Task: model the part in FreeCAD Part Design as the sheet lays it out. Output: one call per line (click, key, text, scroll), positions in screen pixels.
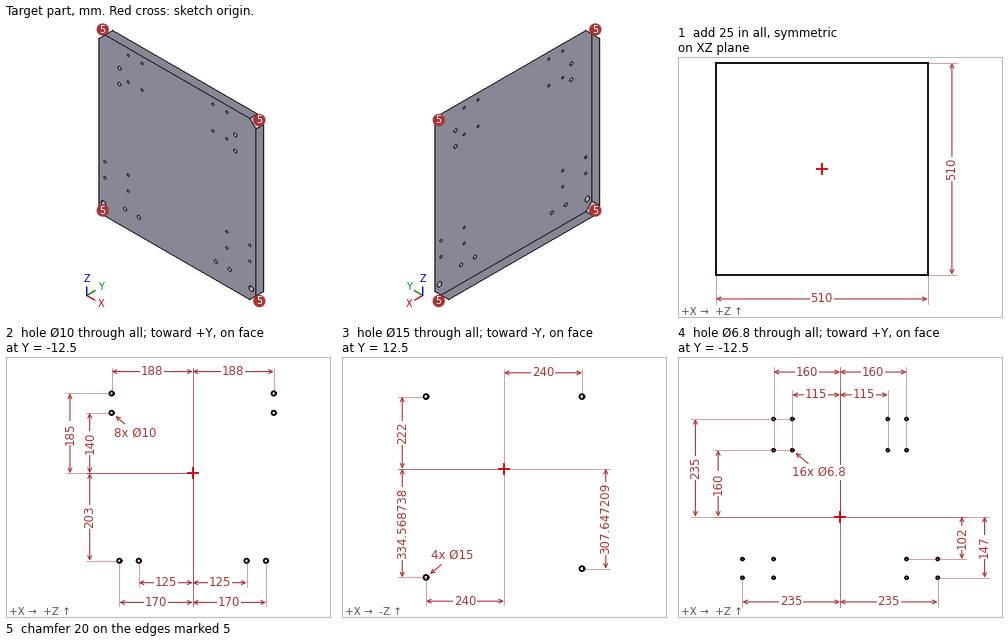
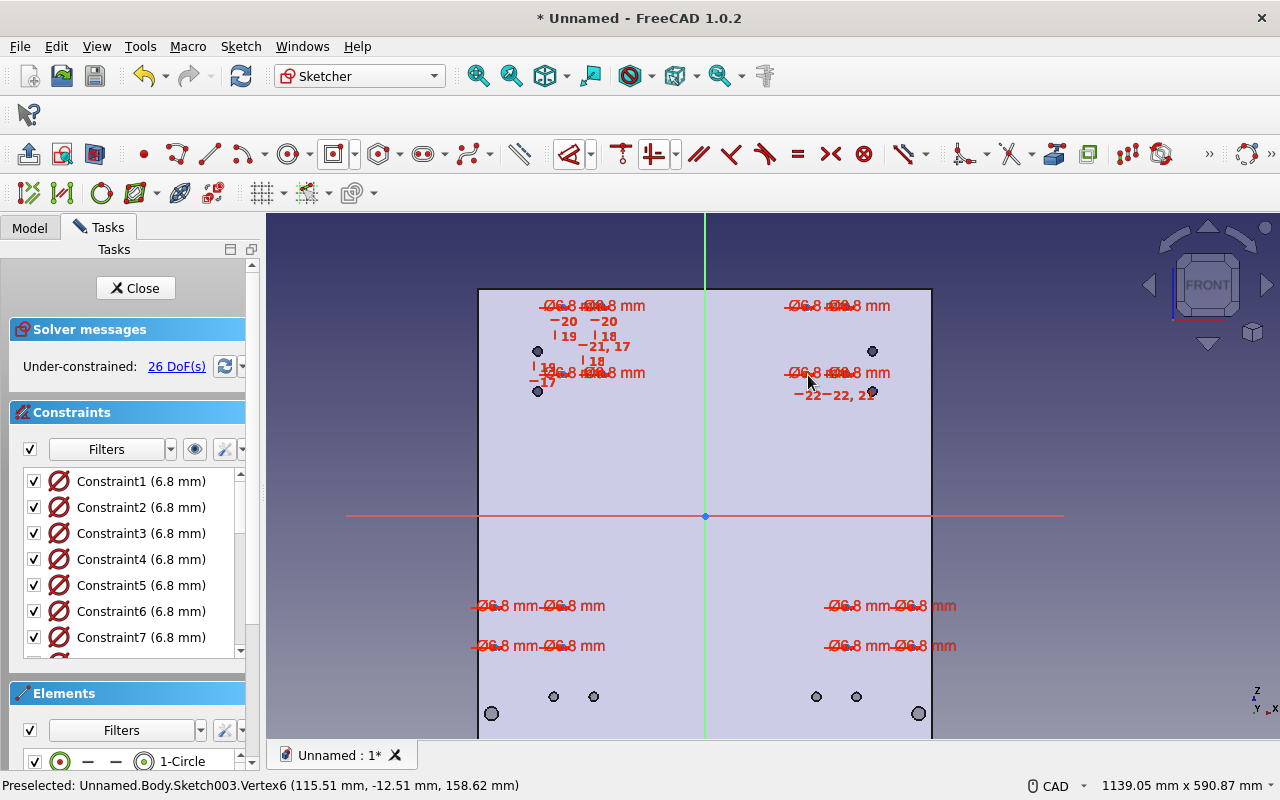
click(808, 308)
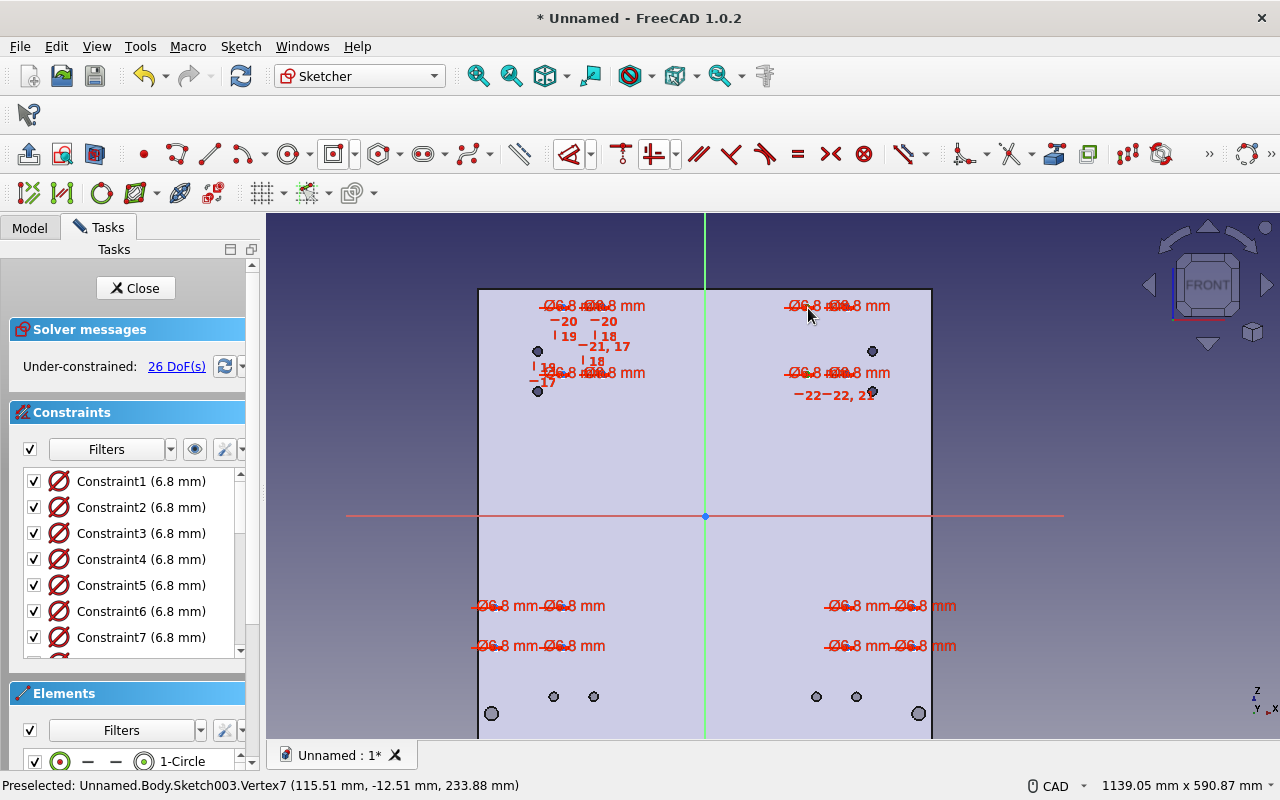
key(v)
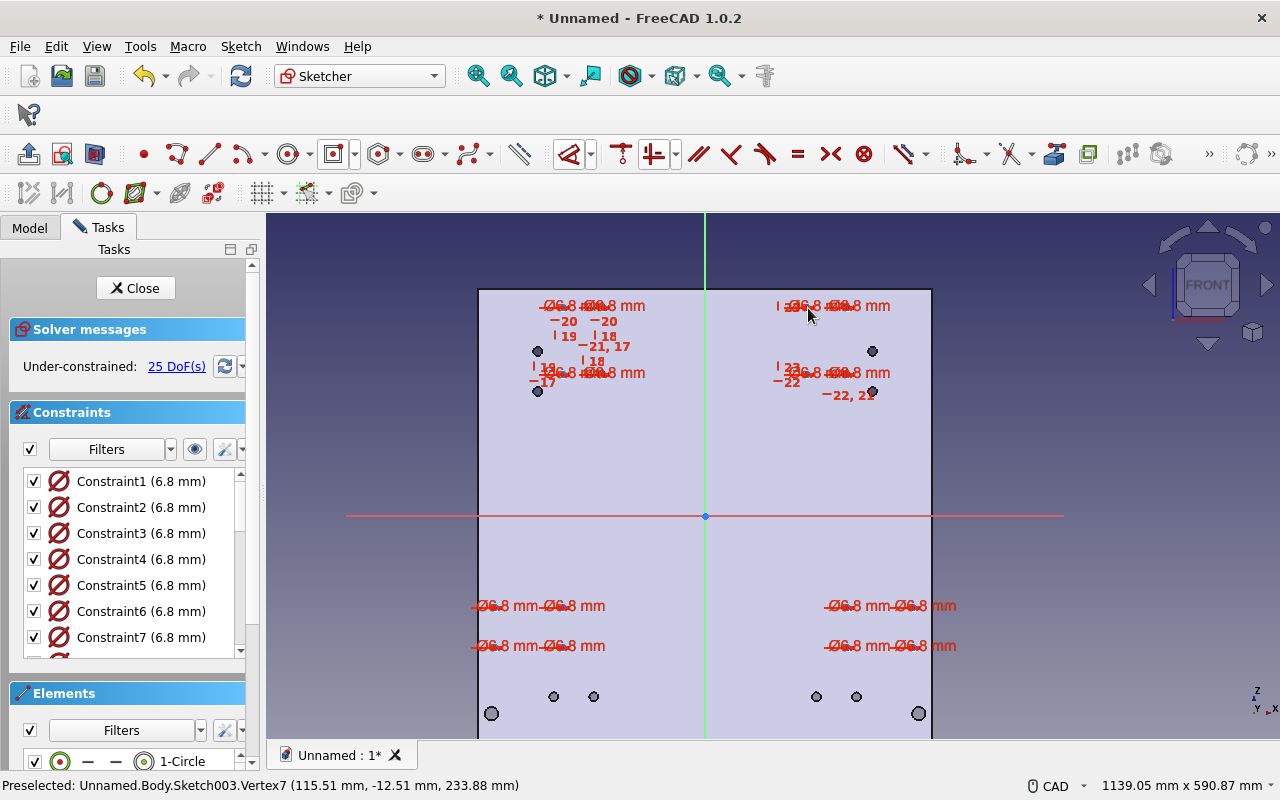
click(603, 308)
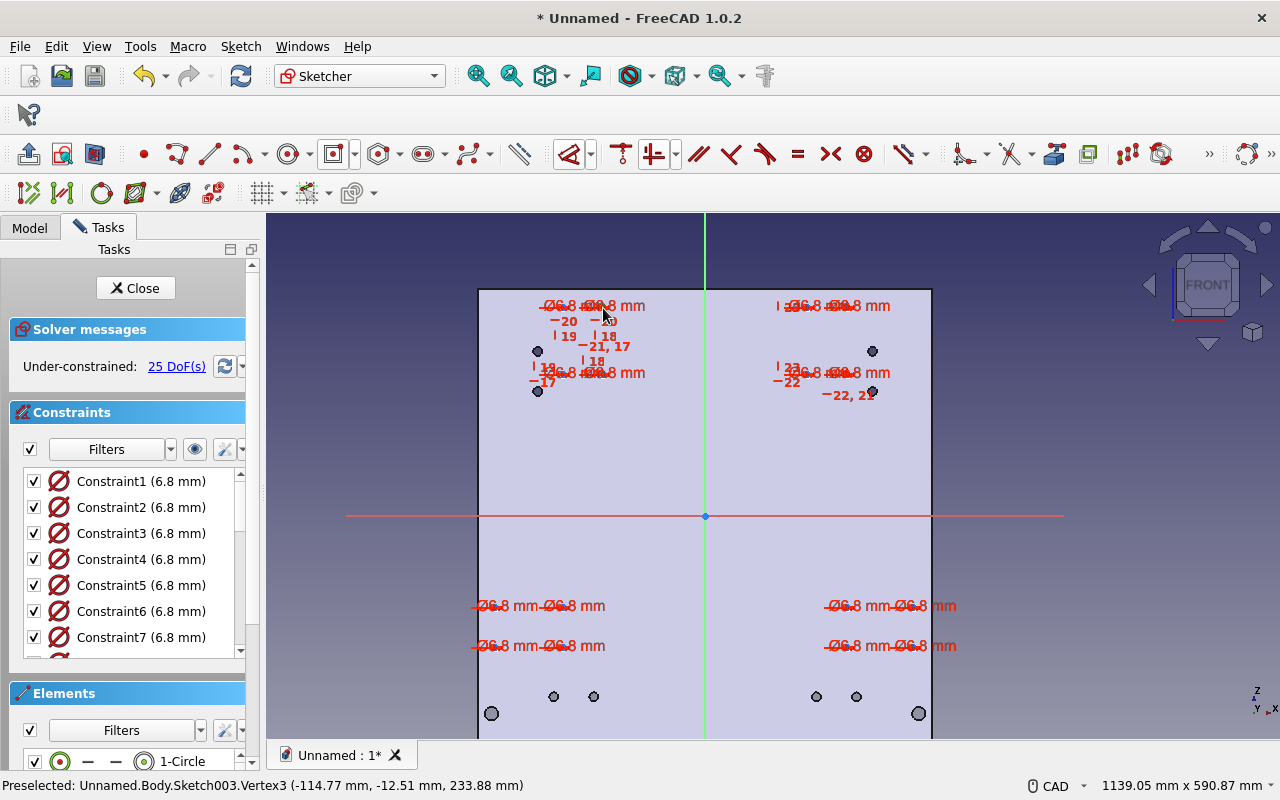
click(808, 308)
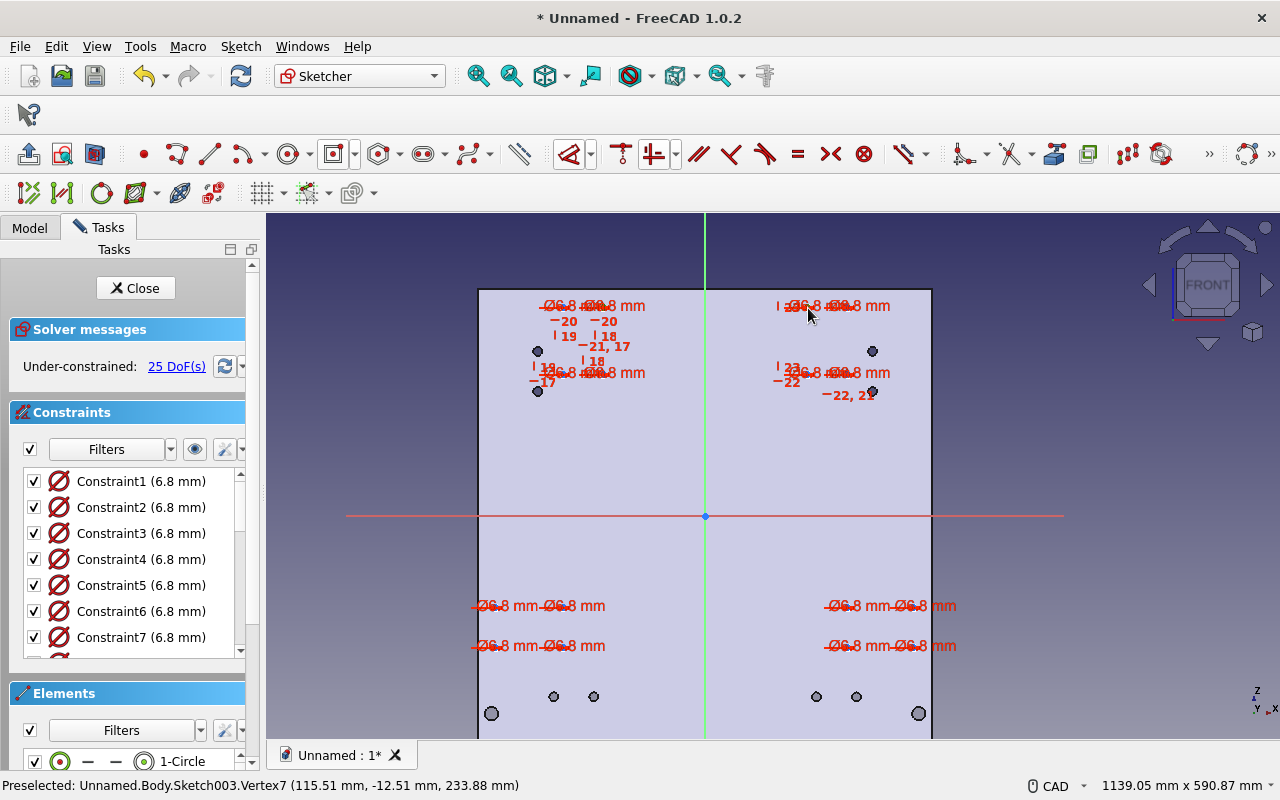
key(h)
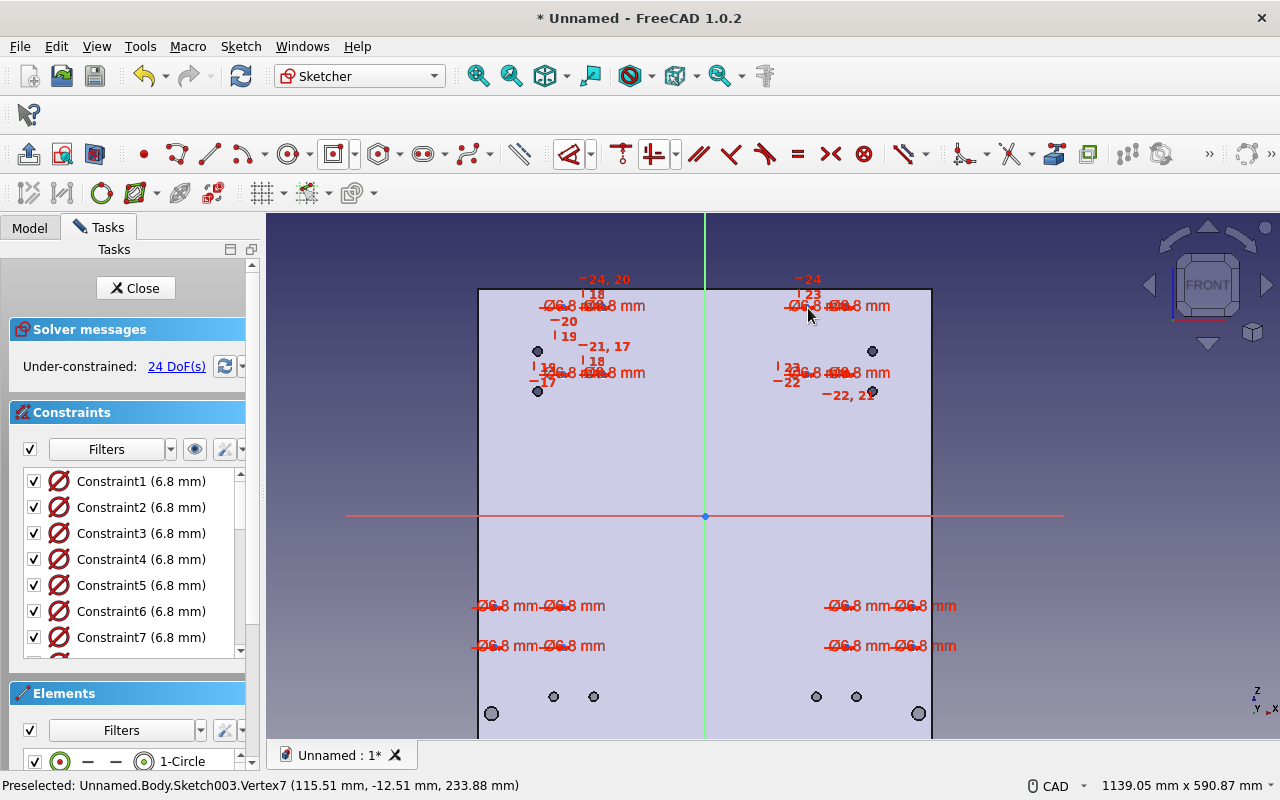
click(848, 375)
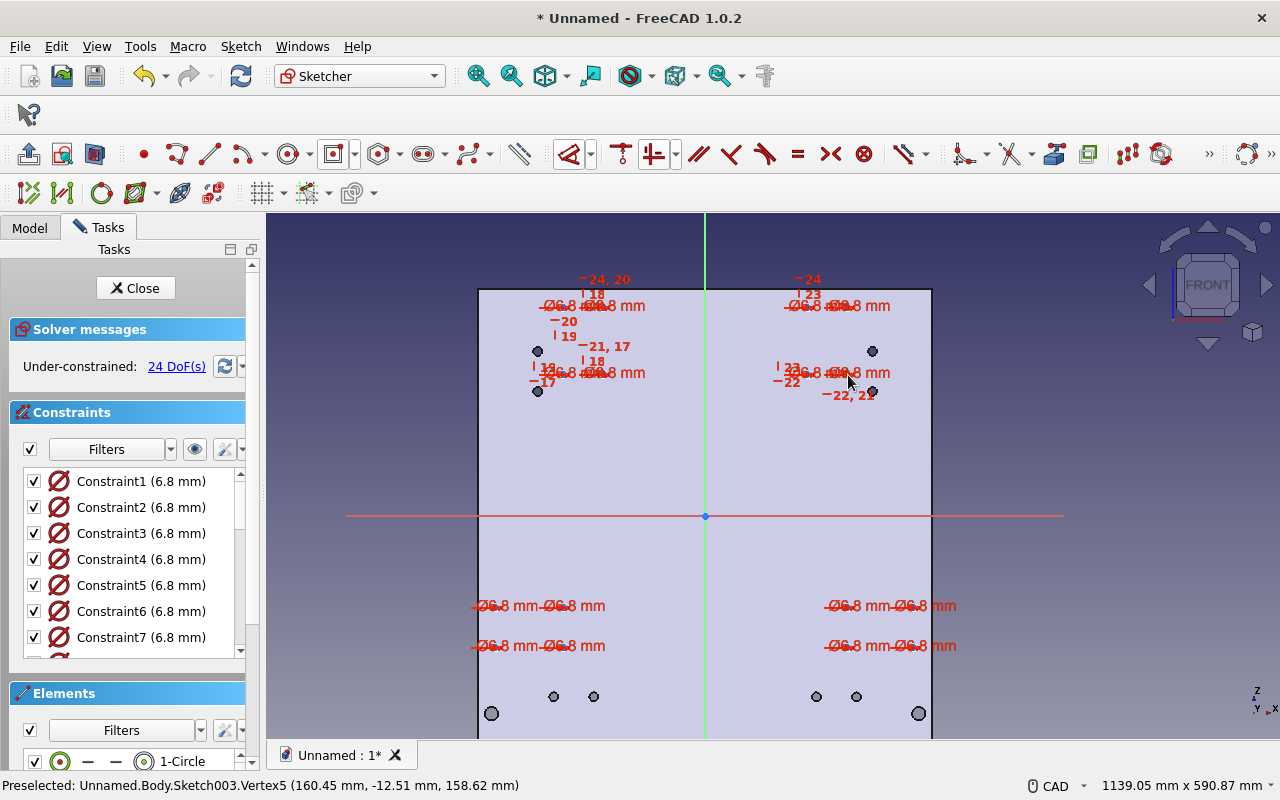
click(848, 308)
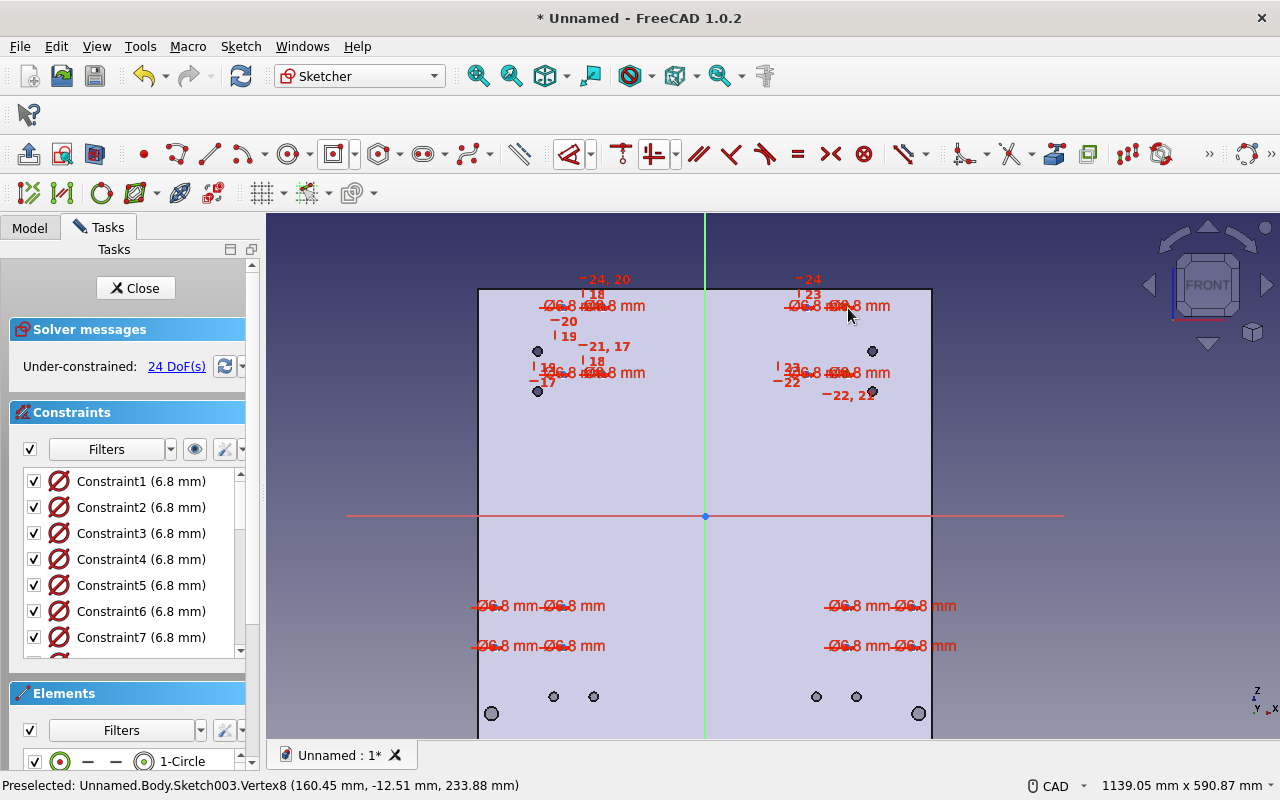
click(676, 154)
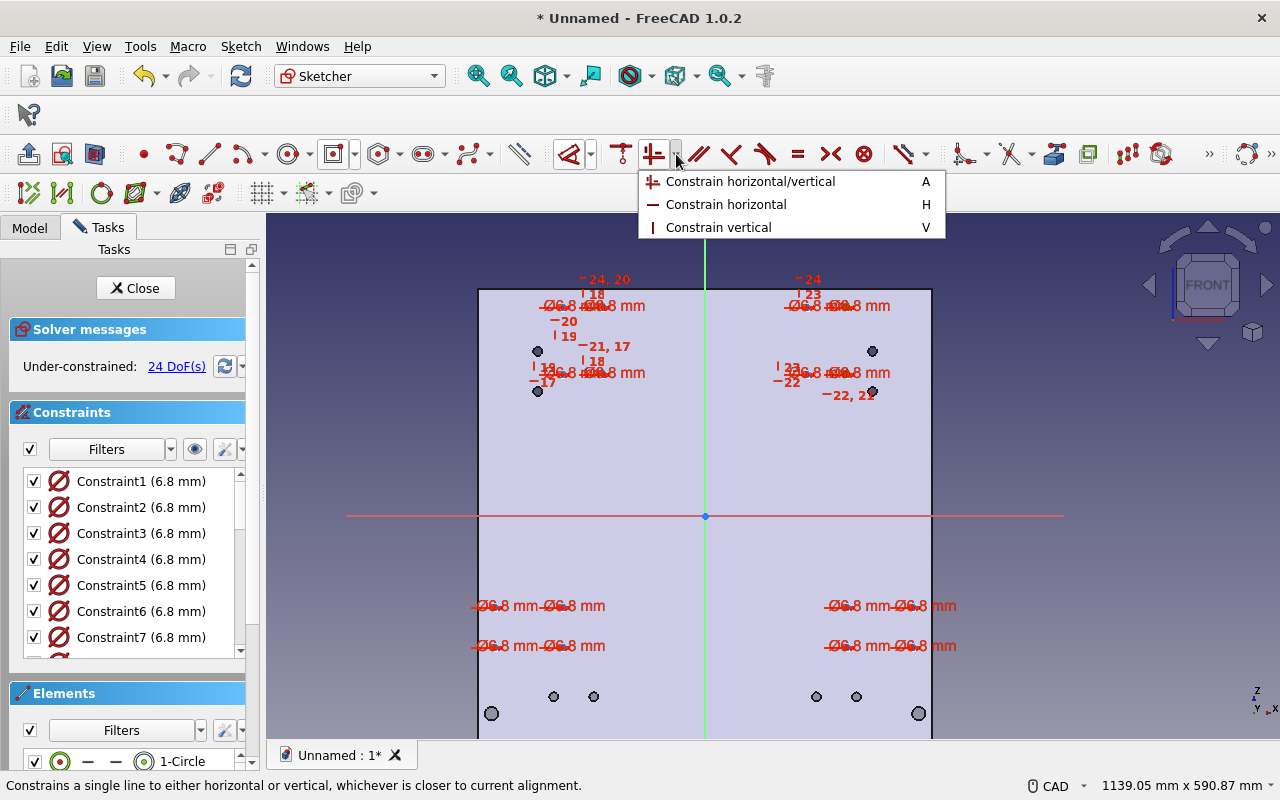
click(792, 228)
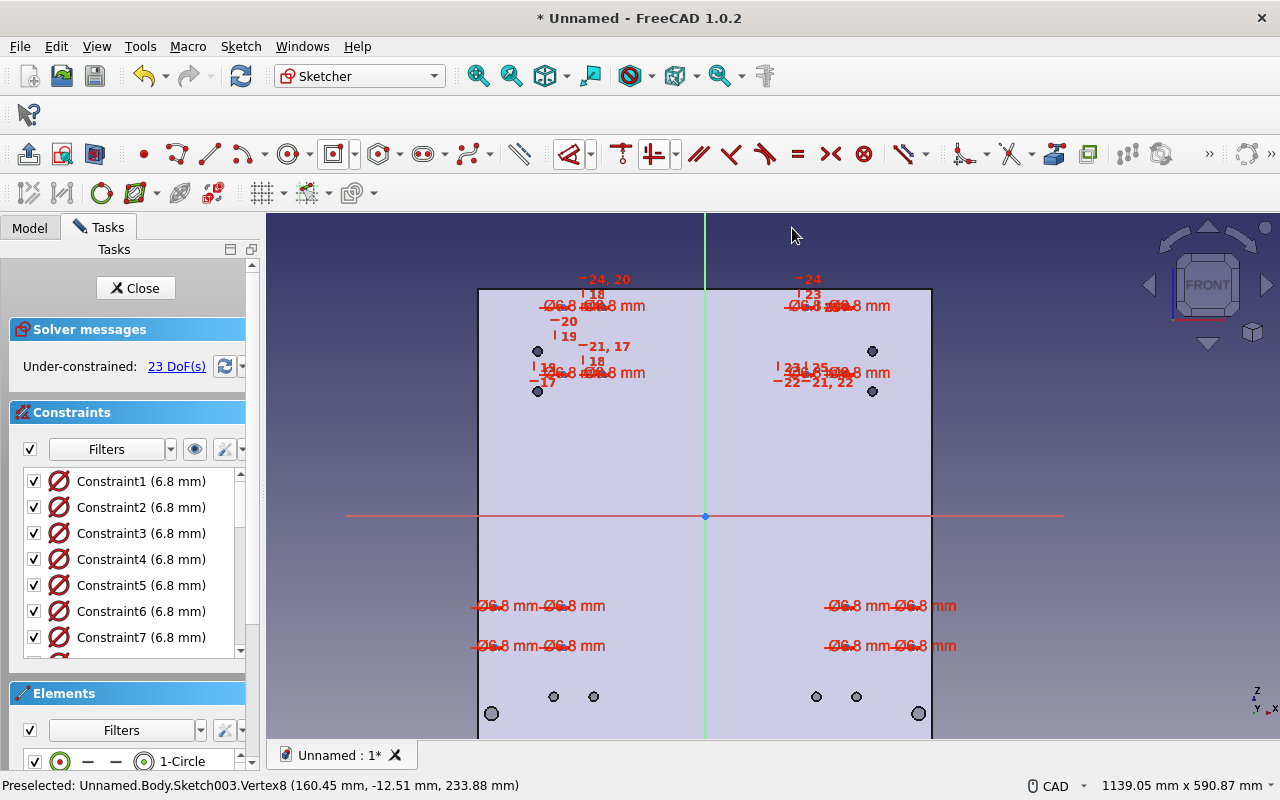
click(808, 308)